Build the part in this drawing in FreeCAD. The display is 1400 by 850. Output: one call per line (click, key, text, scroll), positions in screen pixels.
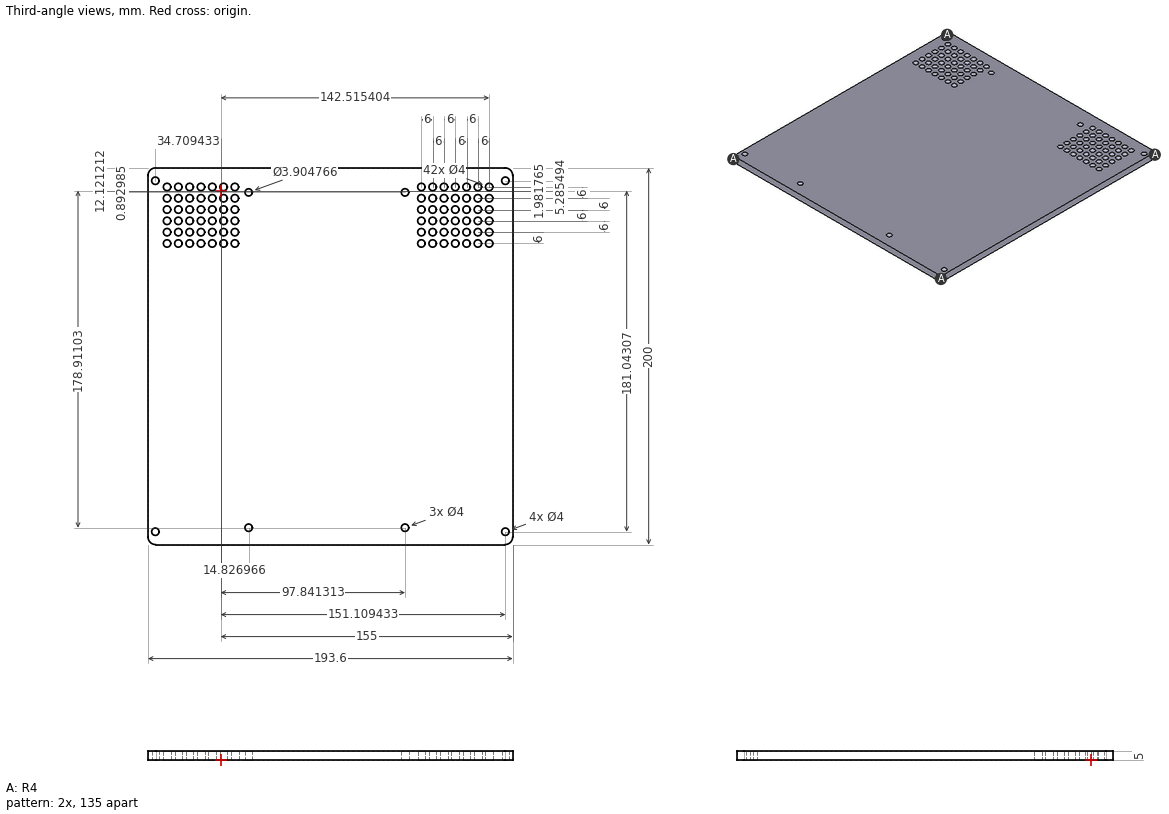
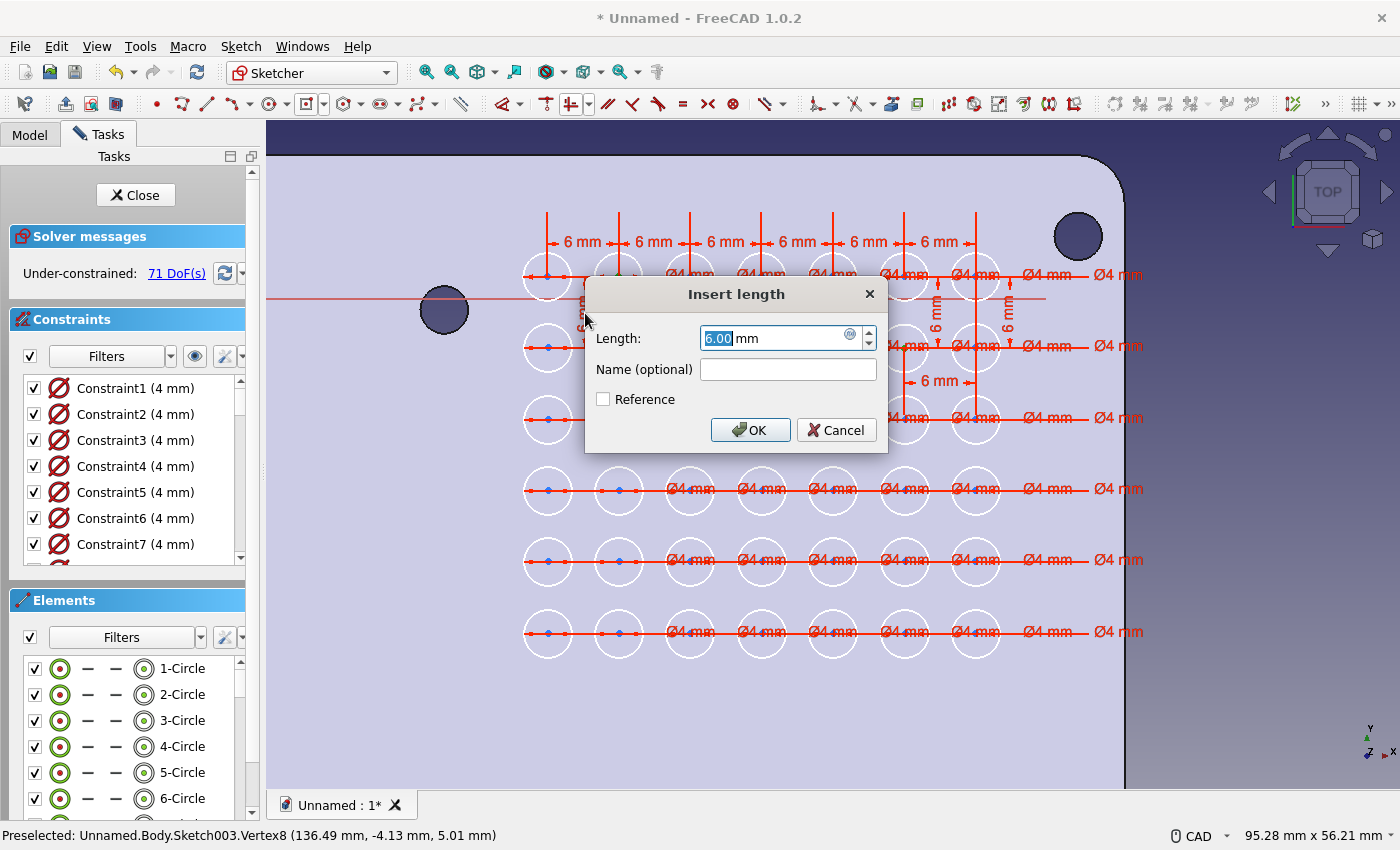
text(6)
key(Return)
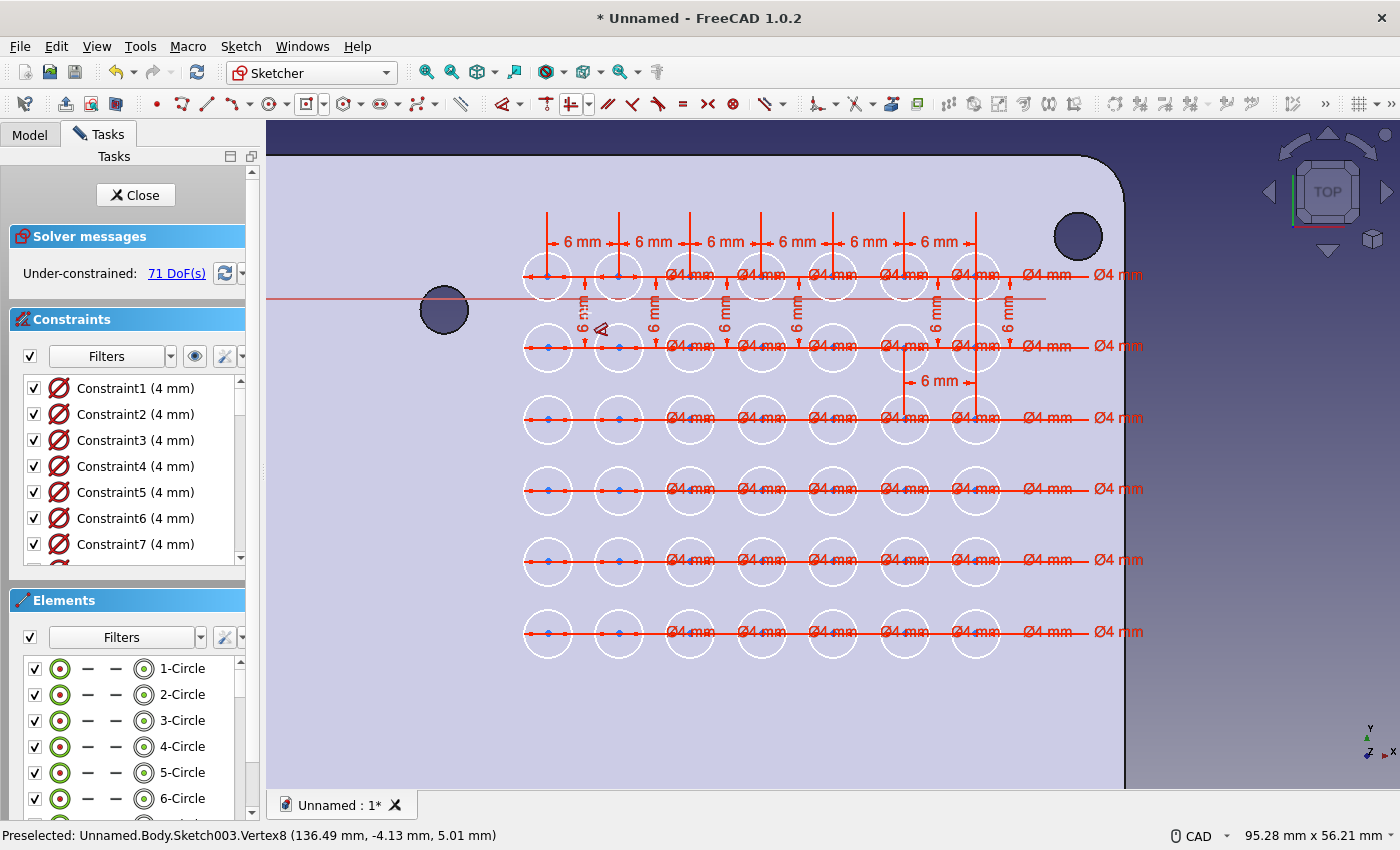
click(904, 348)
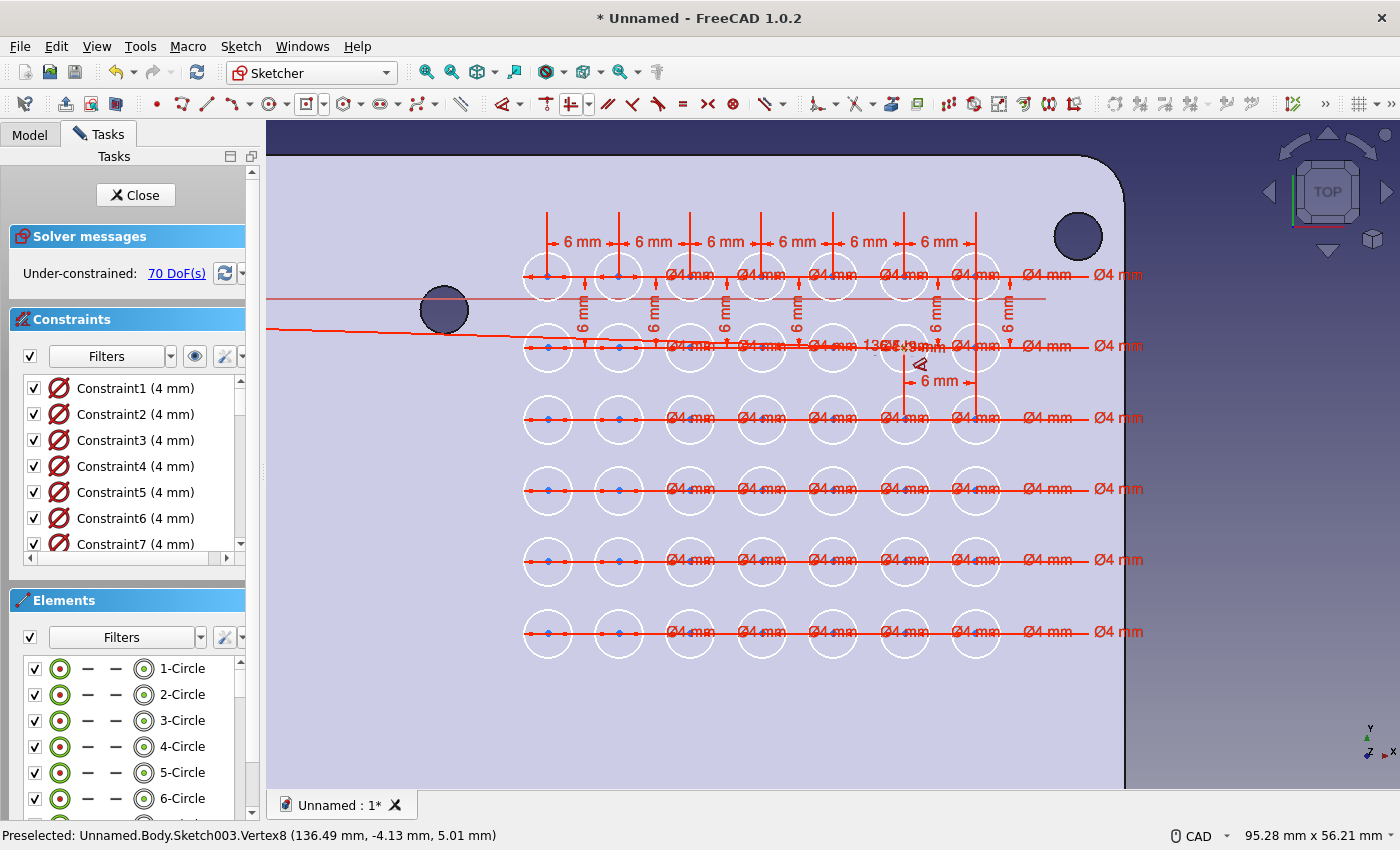
click(833, 348)
click(869, 382)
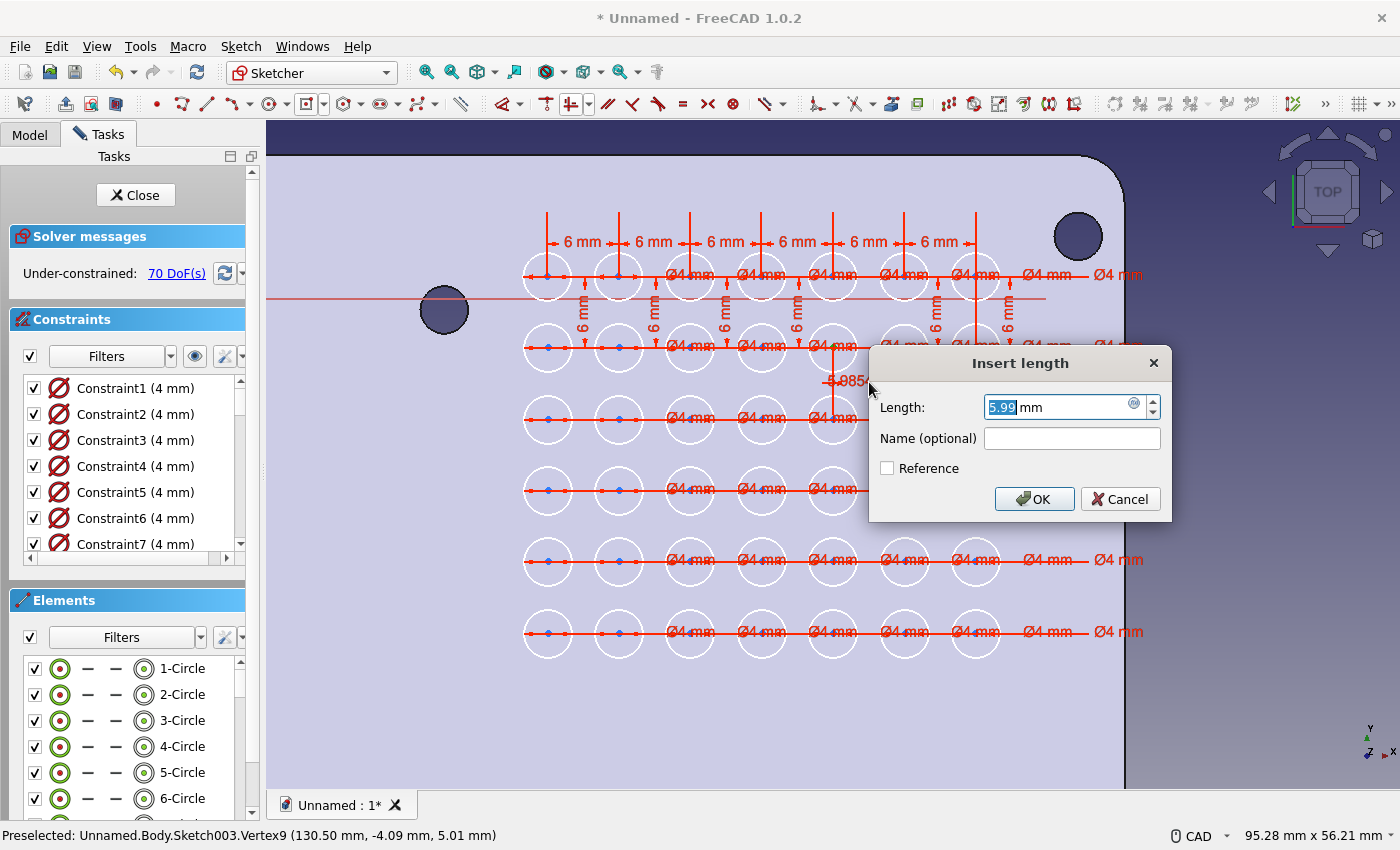
text(6)
key(Return)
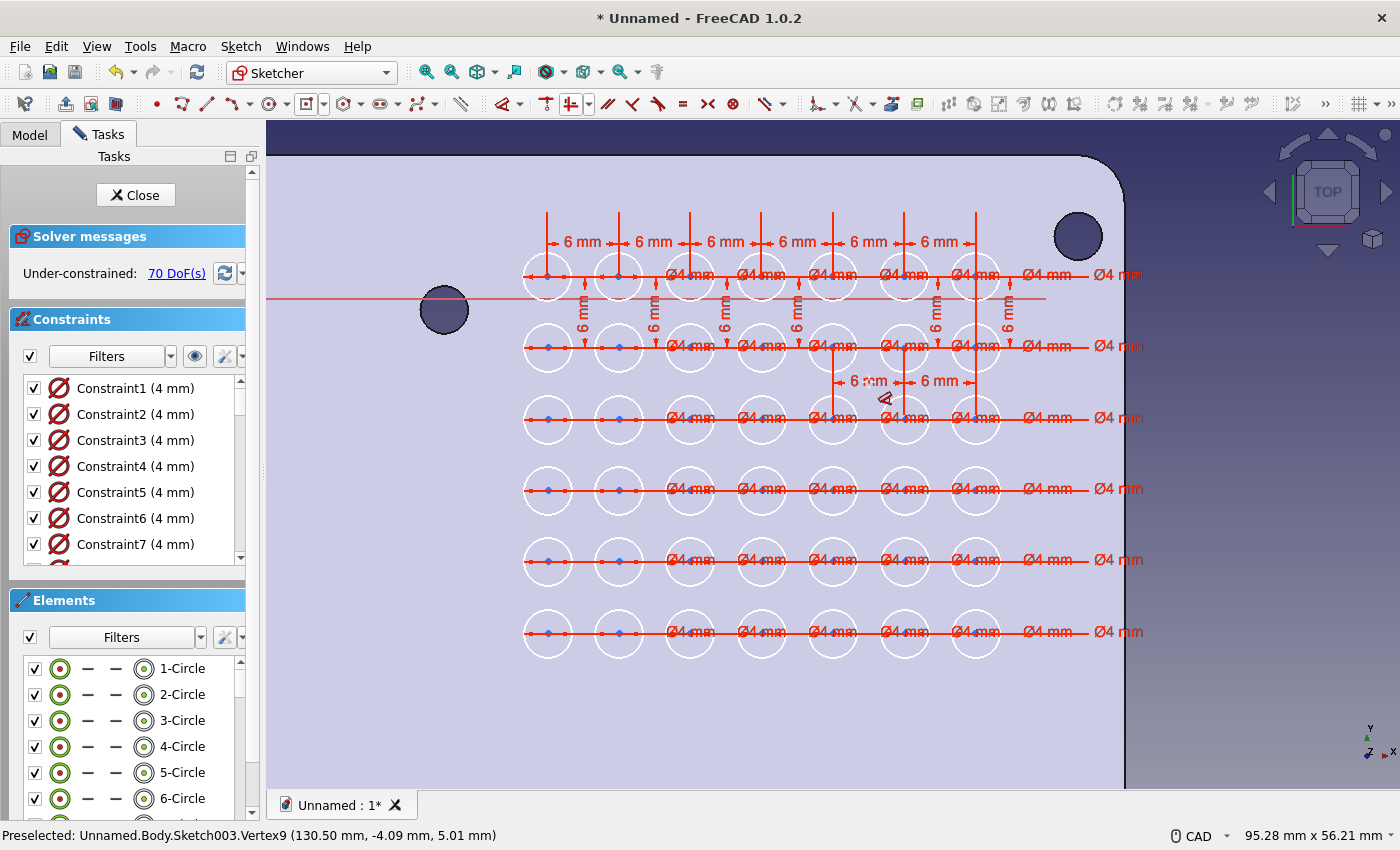
click(833, 277)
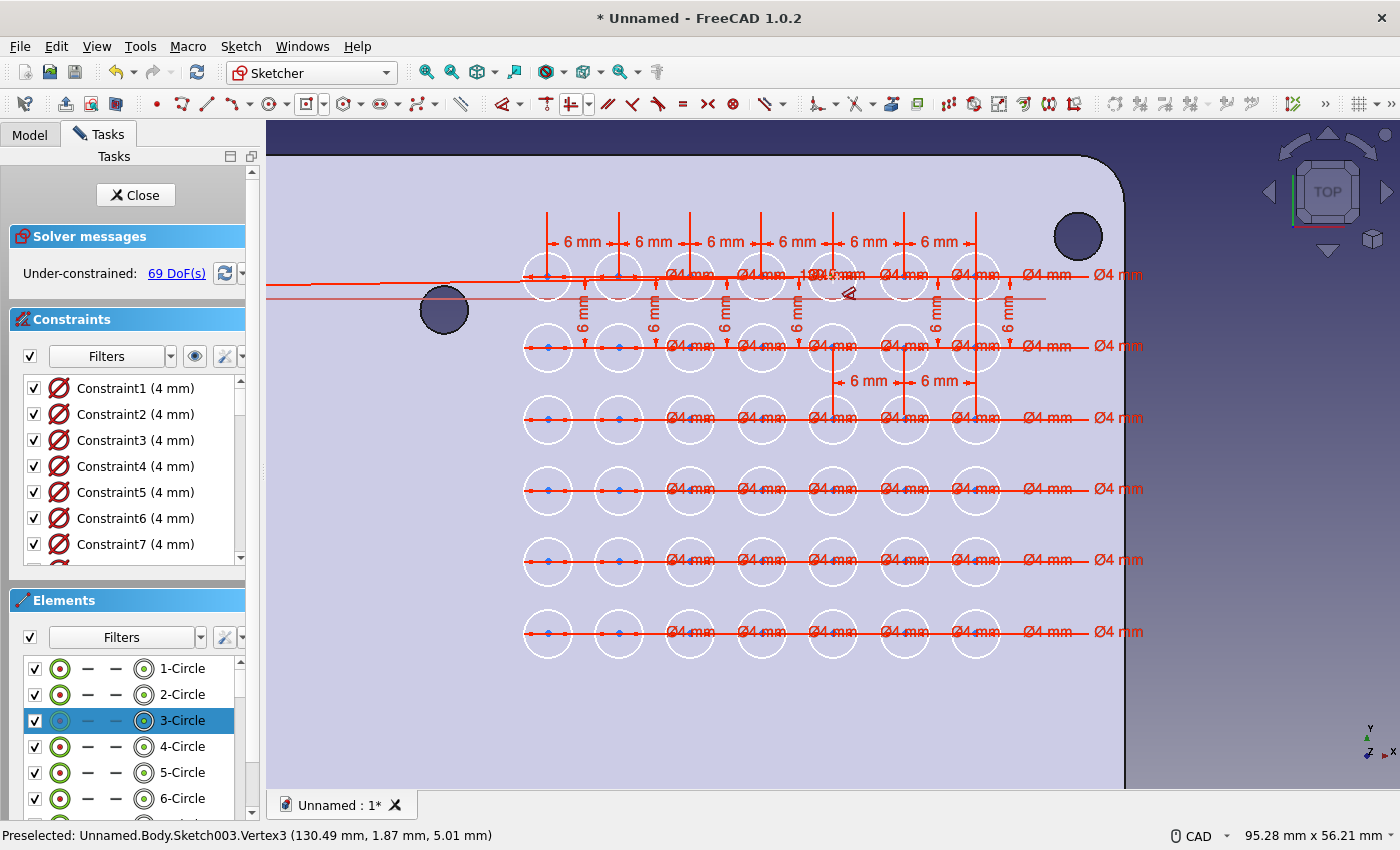
click(833, 348)
click(1013, 337)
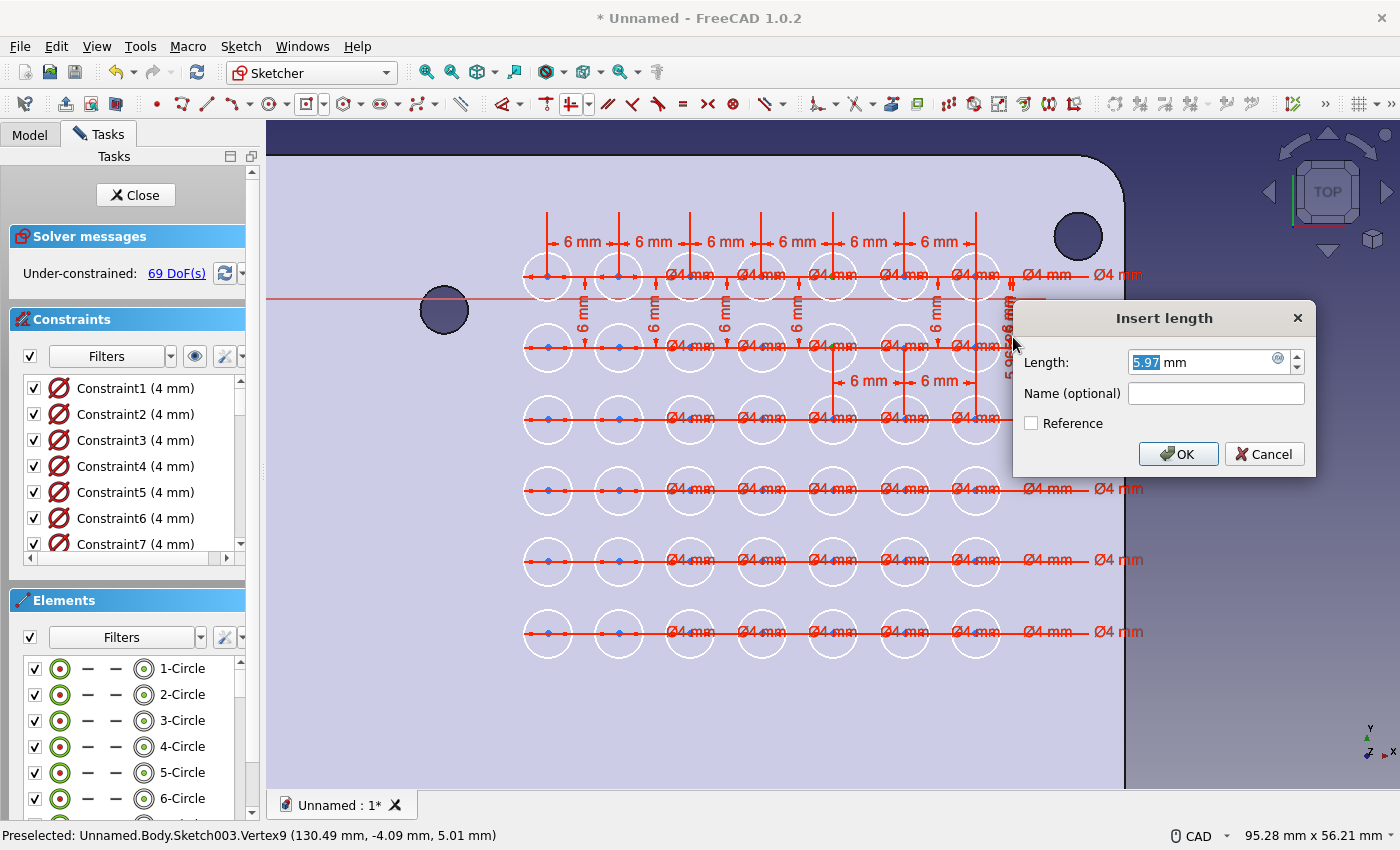
text(6)
key(Return)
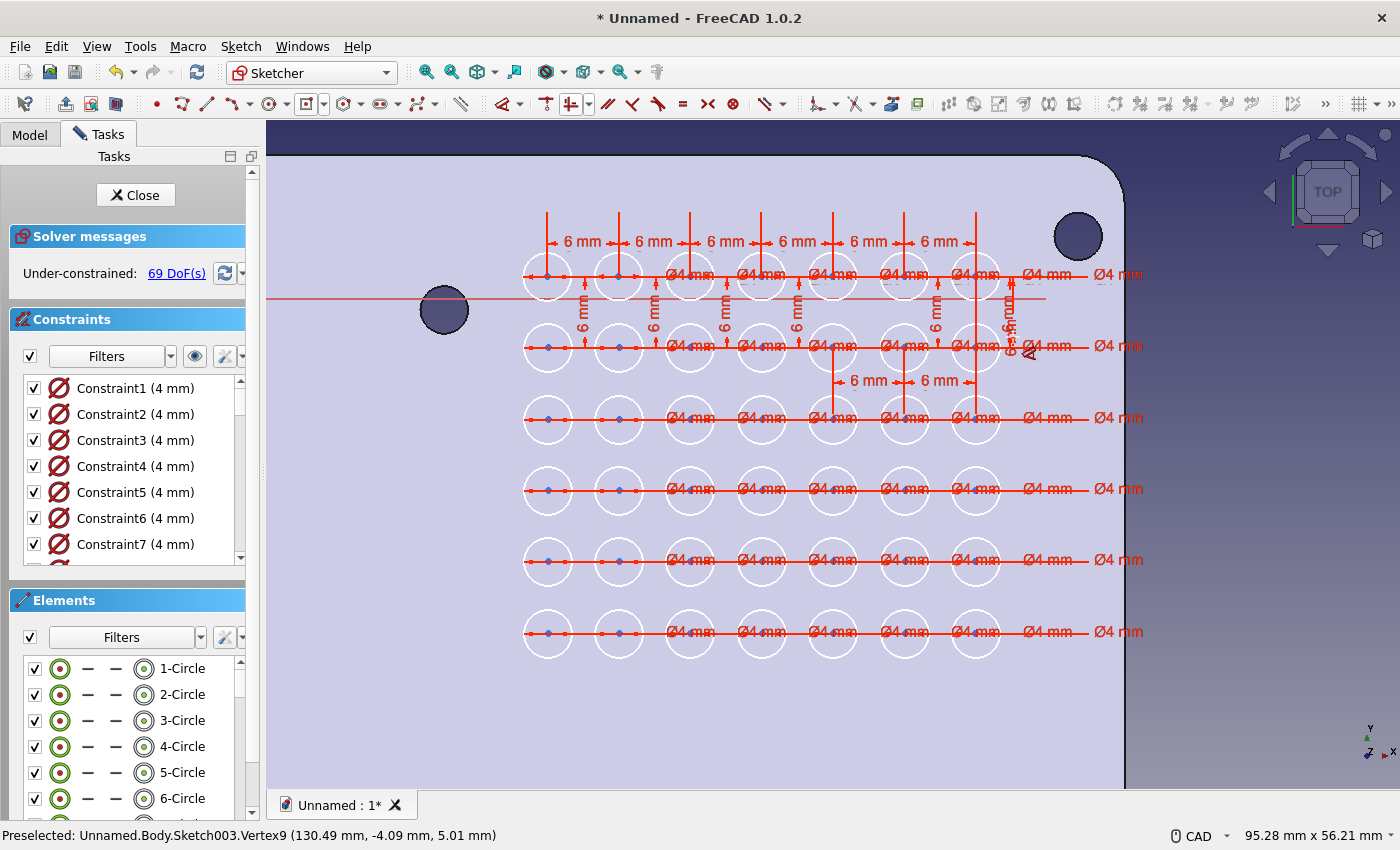
click(833, 348)